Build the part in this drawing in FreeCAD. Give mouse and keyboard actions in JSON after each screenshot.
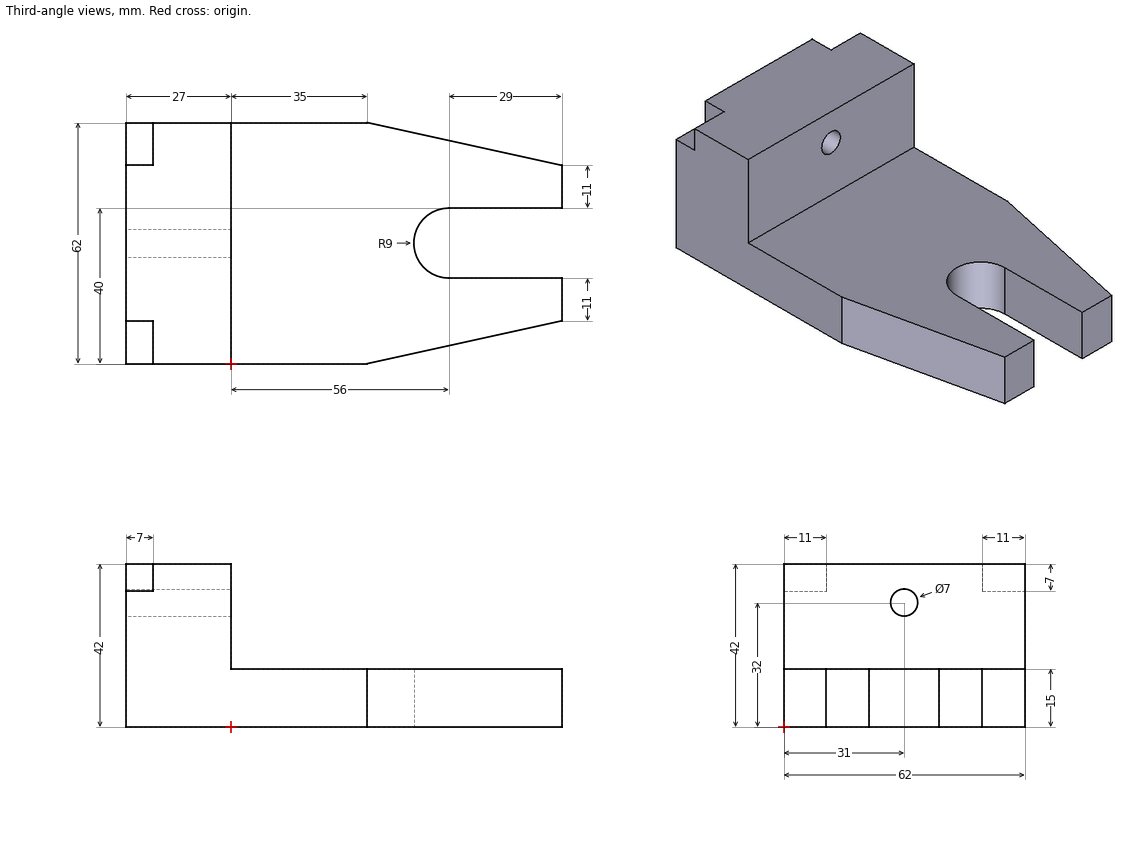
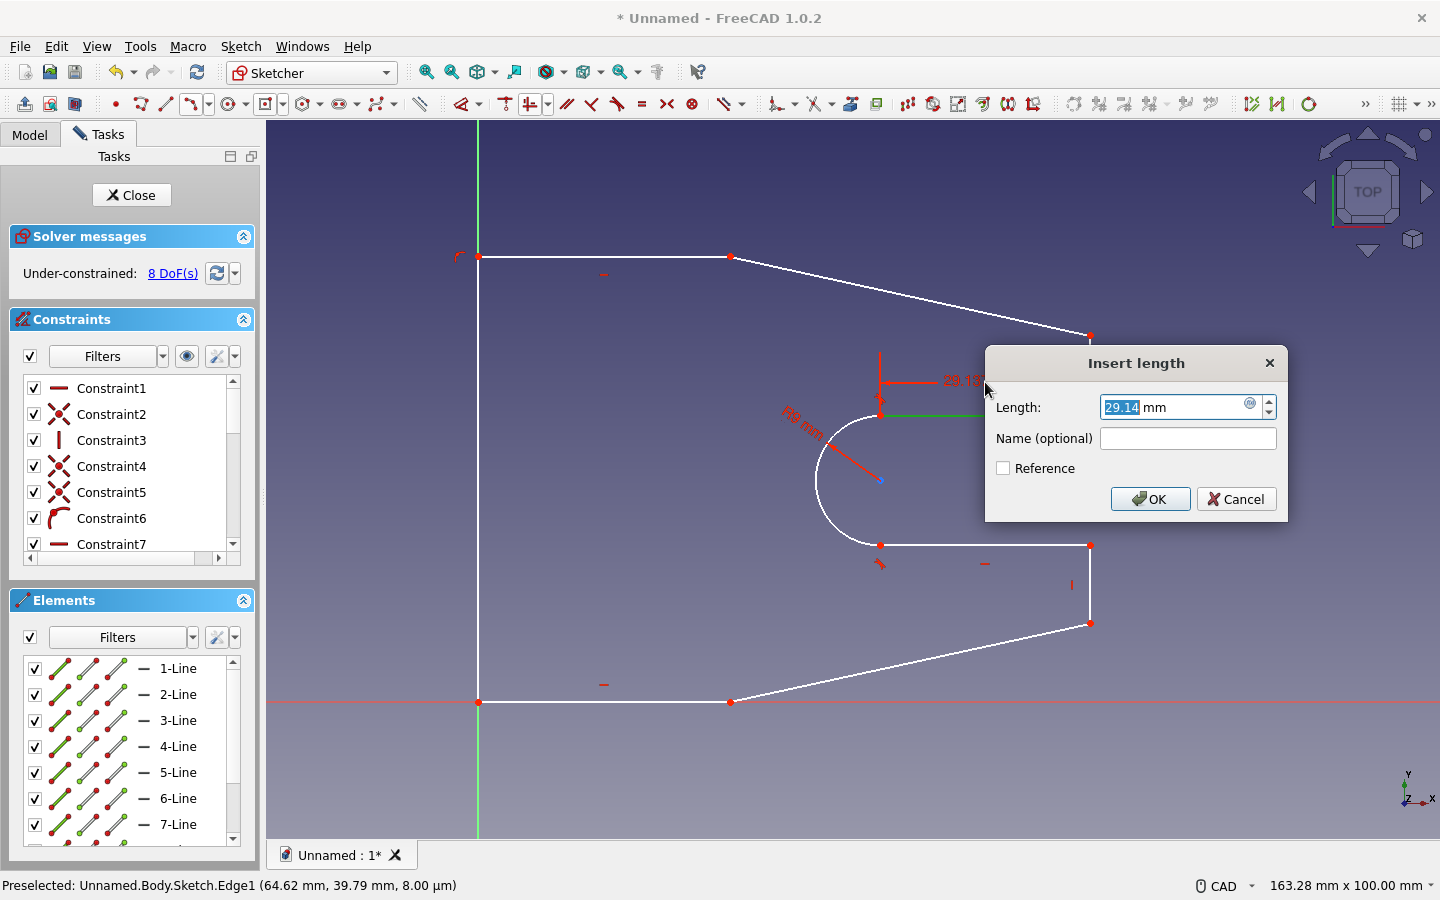
{"action": "type", "text": "29"}
{"action": "key", "text": "Return"}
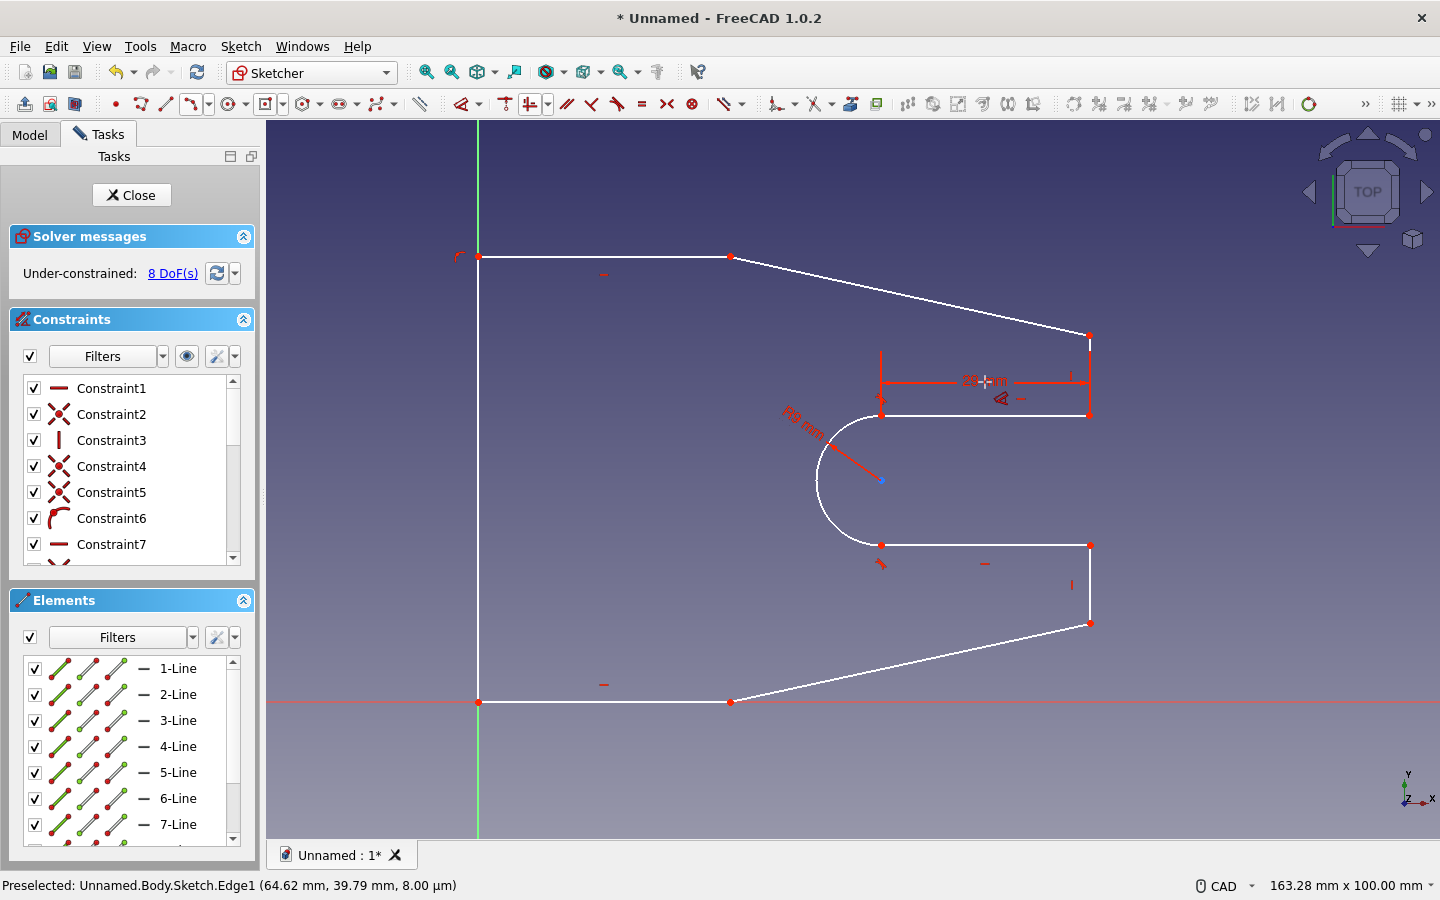
{"action": "left_click", "coordinate": [1090, 392]}
{"action": "left_click", "coordinate": [1124, 376]}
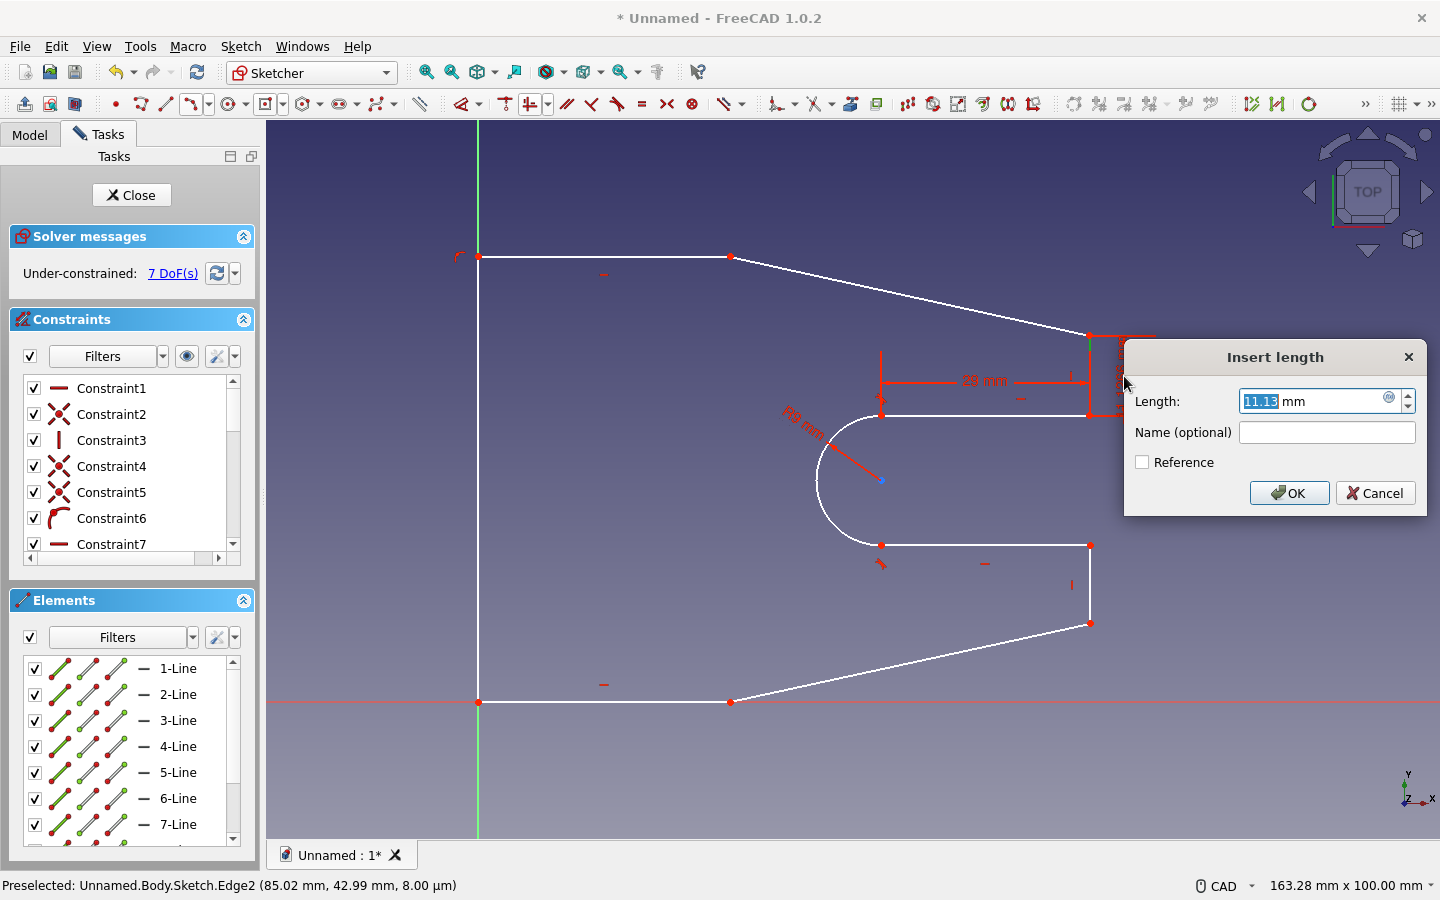
{"action": "type", "text": "11"}
{"action": "key", "text": "Return"}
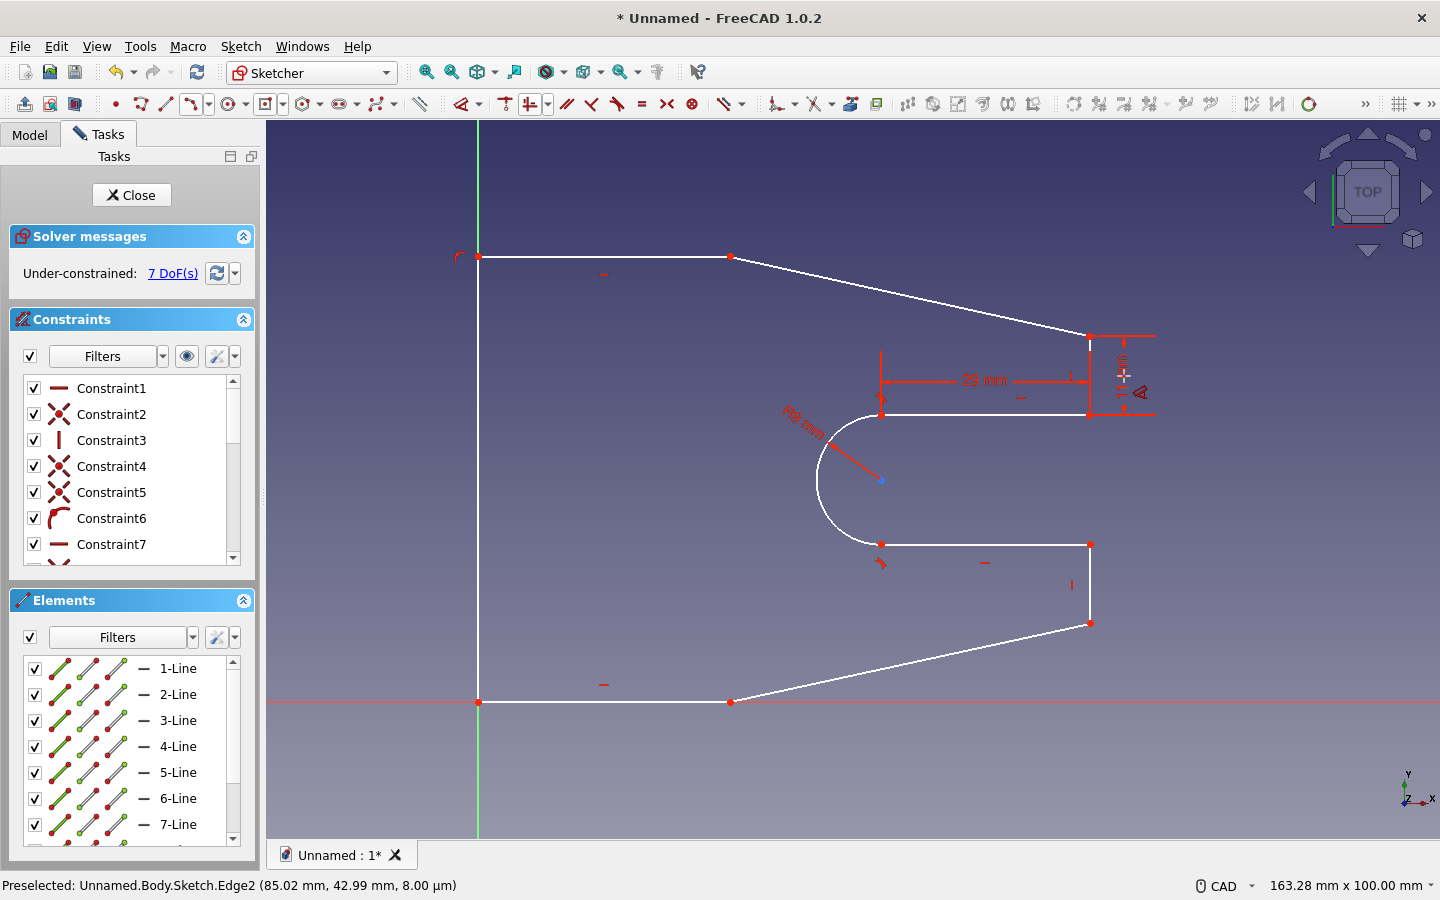
{"action": "left_click", "coordinate": [655, 257]}
{"action": "left_click", "coordinate": [604, 223]}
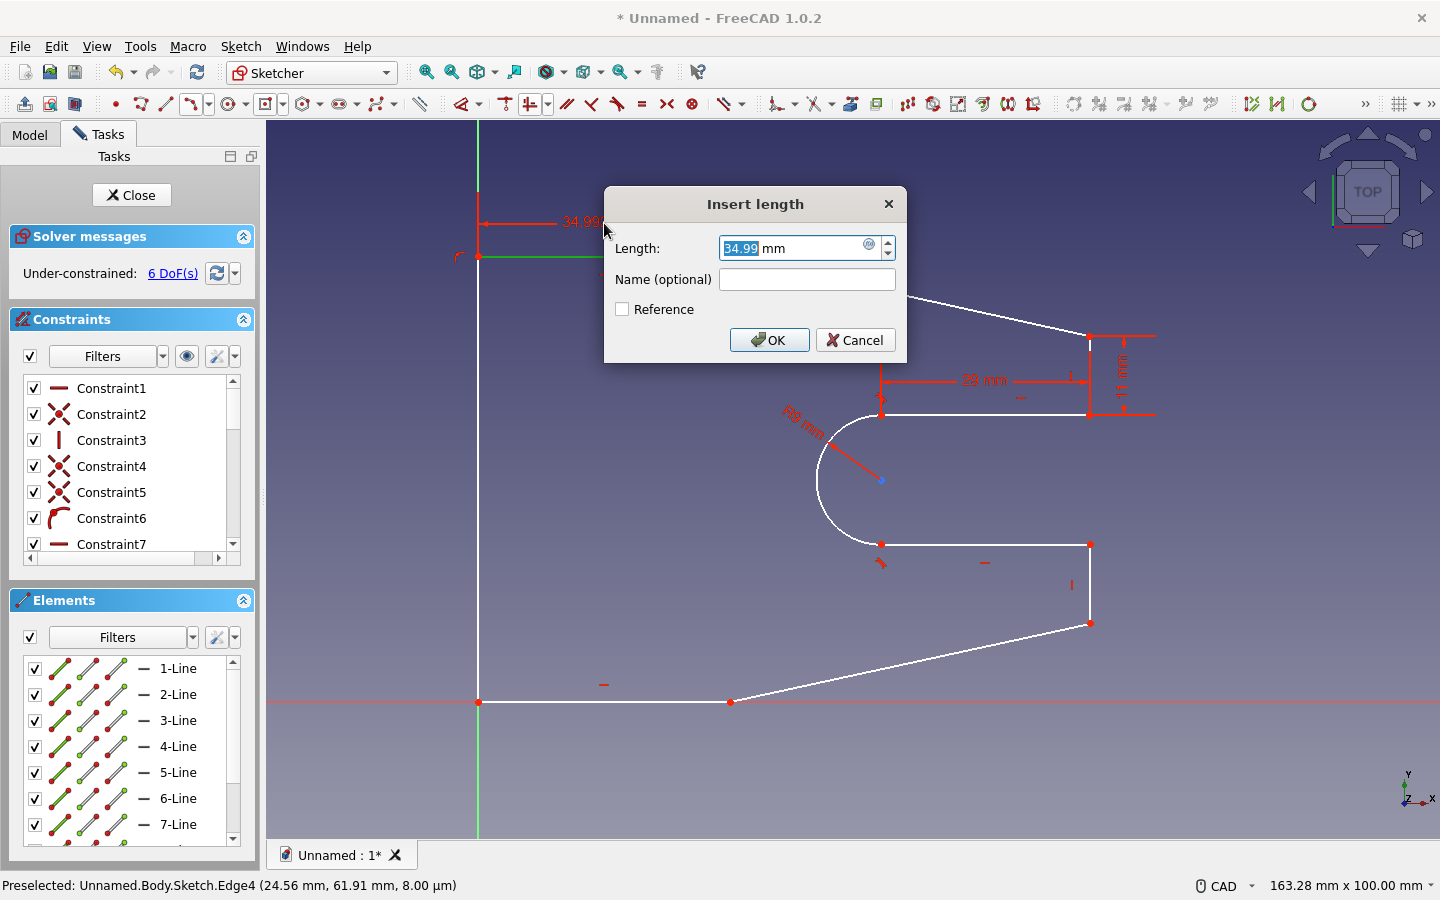
{"action": "type", "text": "35"}
{"action": "key", "text": "Return"}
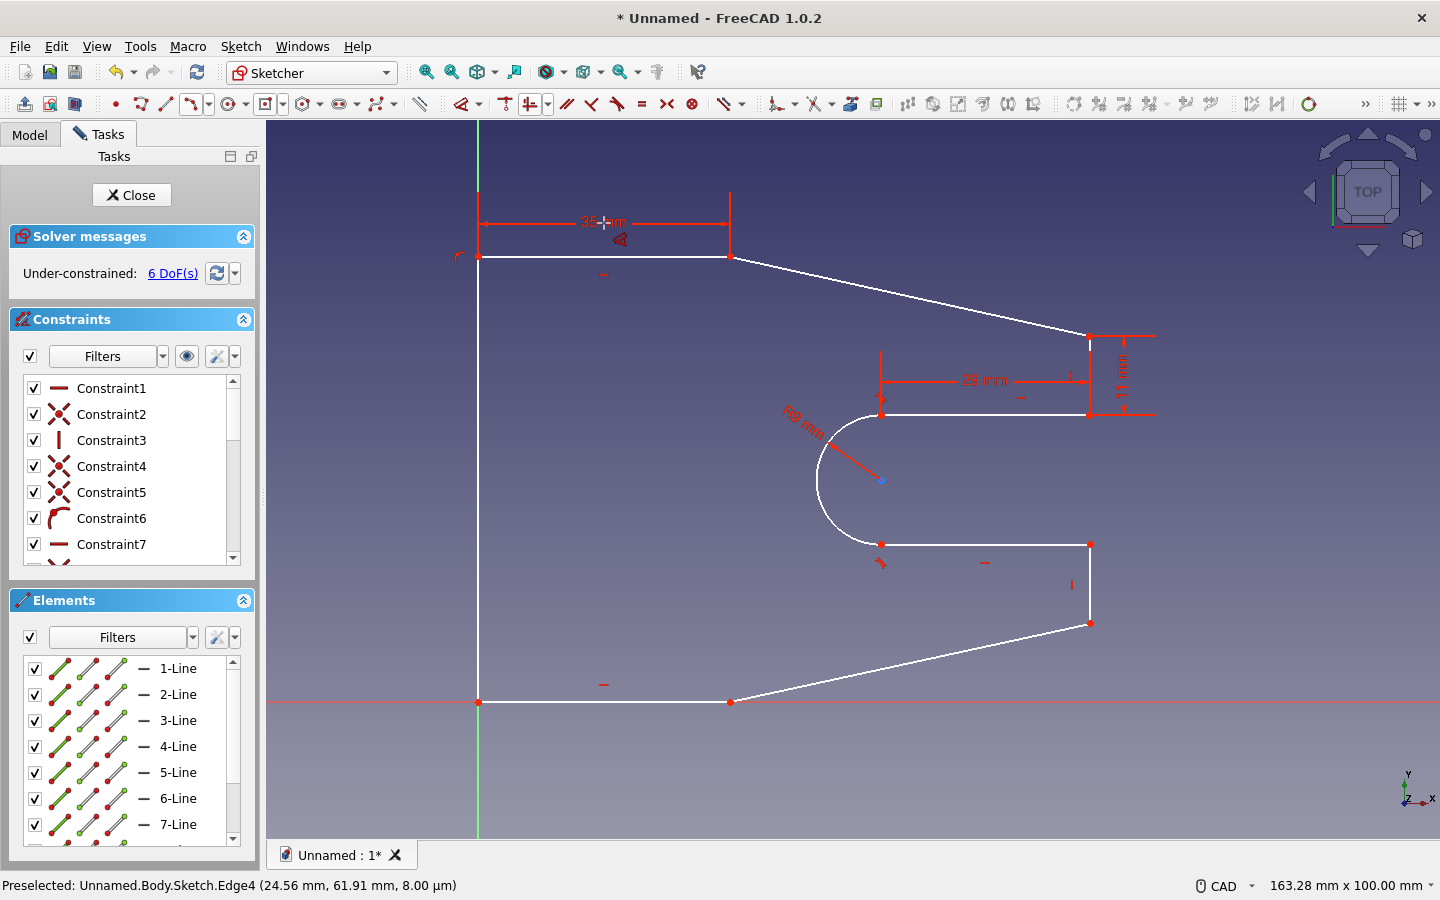
{"action": "left_click", "coordinate": [478, 391]}
{"action": "left_click", "coordinate": [444, 480]}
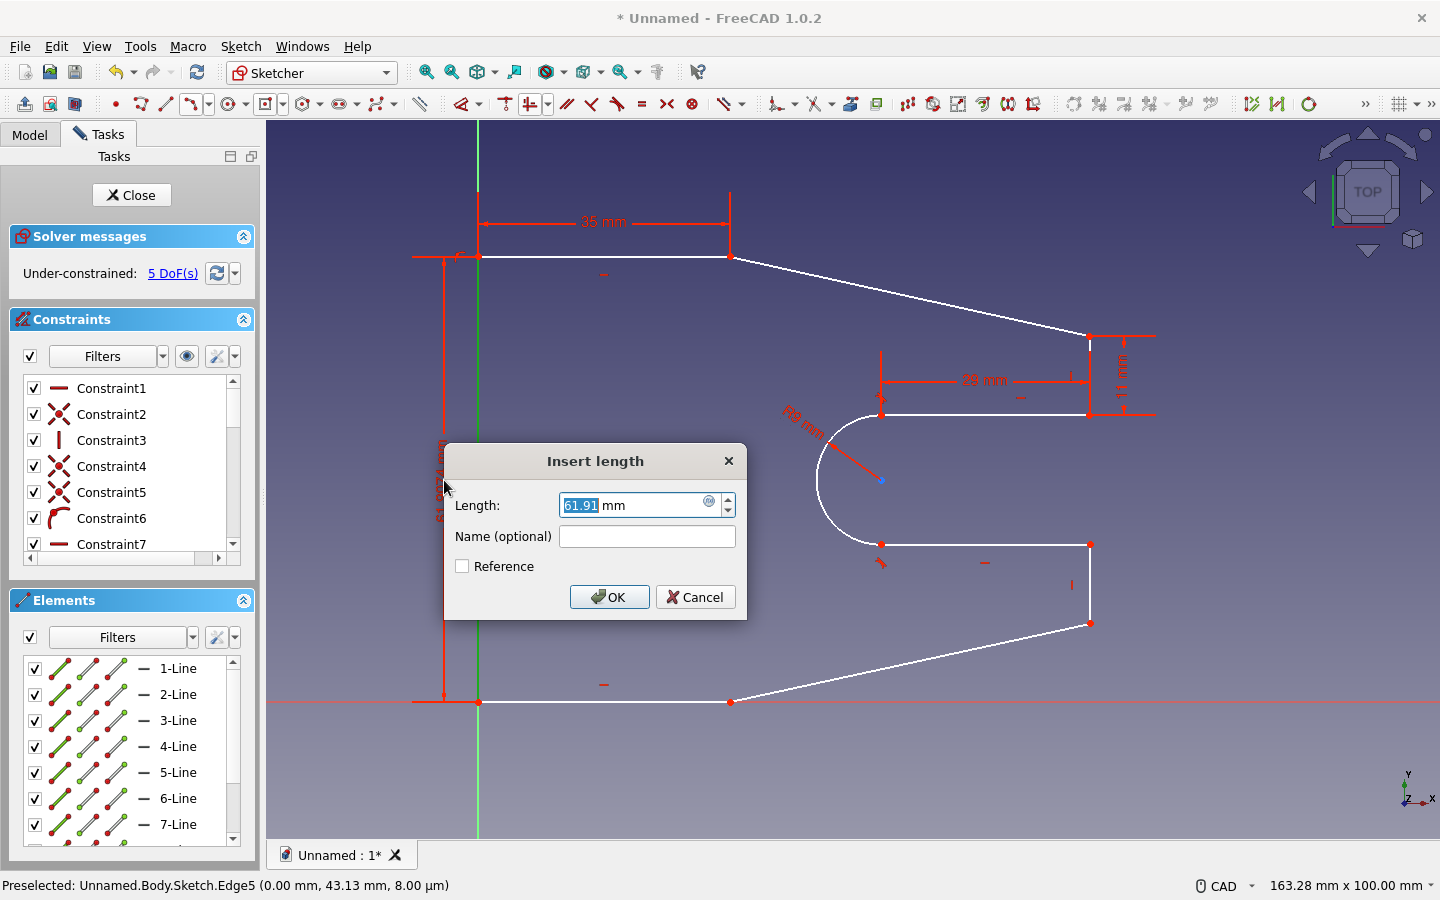
{"action": "type", "text": "62"}
{"action": "key", "text": "Return"}